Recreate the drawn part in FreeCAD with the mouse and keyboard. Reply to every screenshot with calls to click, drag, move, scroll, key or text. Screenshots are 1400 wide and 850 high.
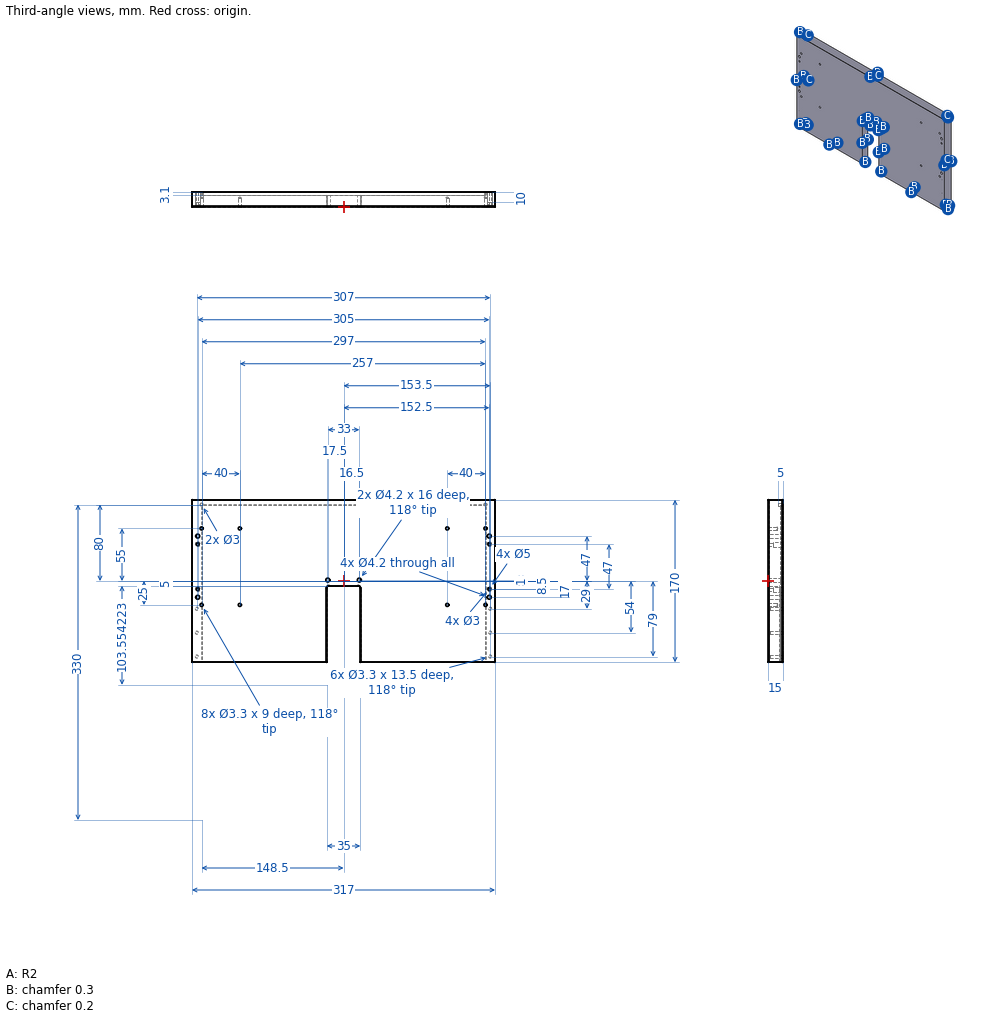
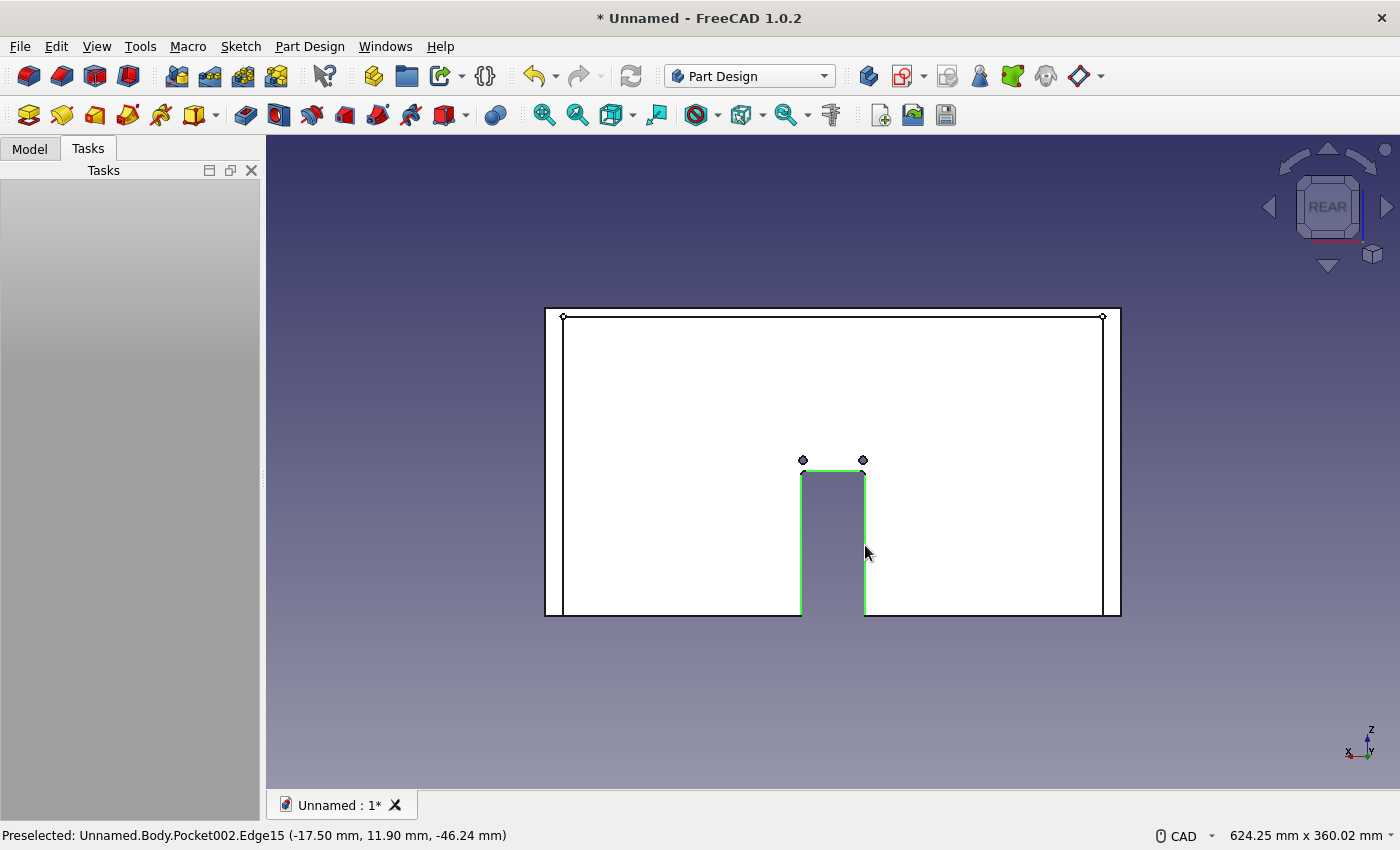
key(6)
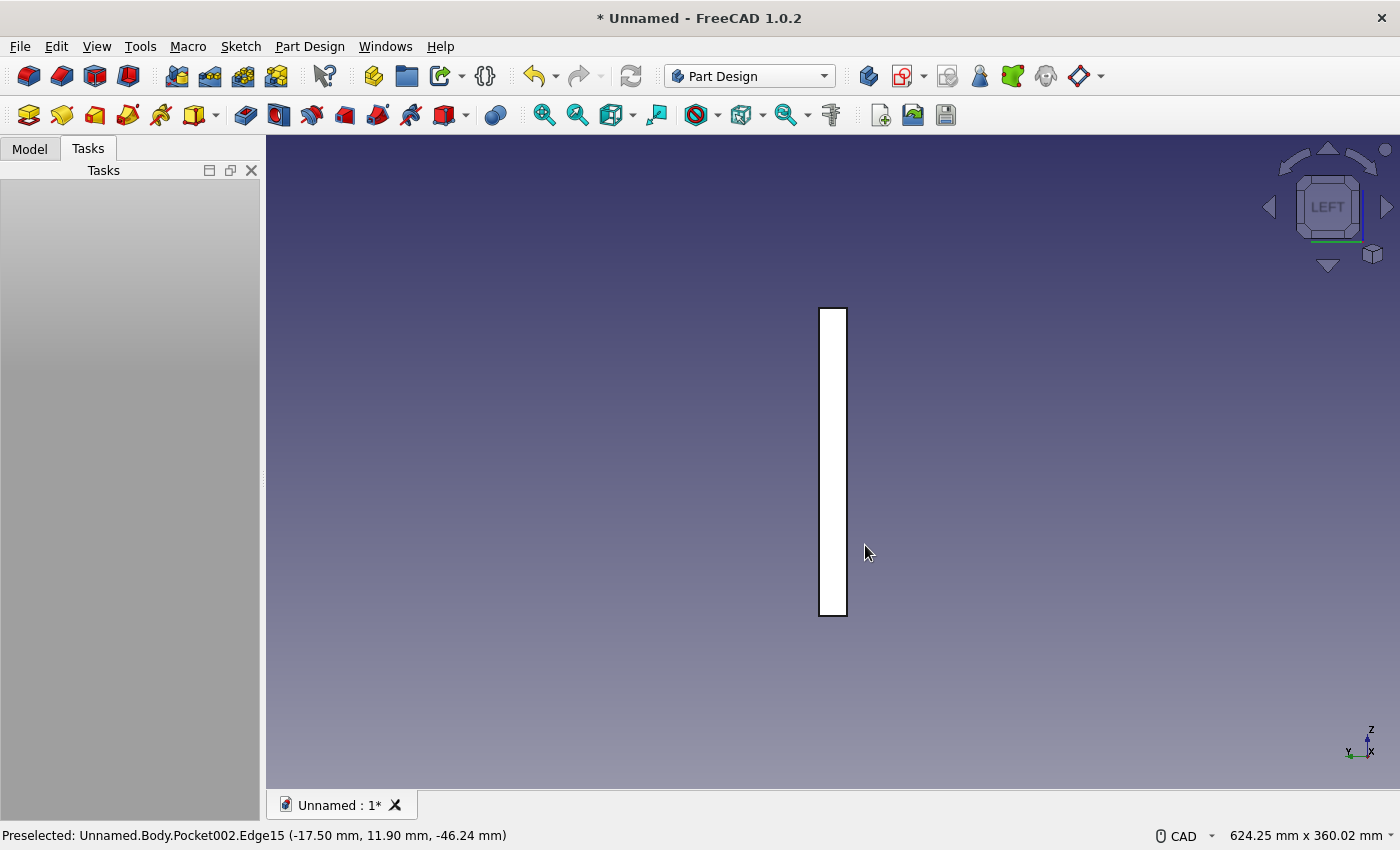
click(833, 329, ctrl)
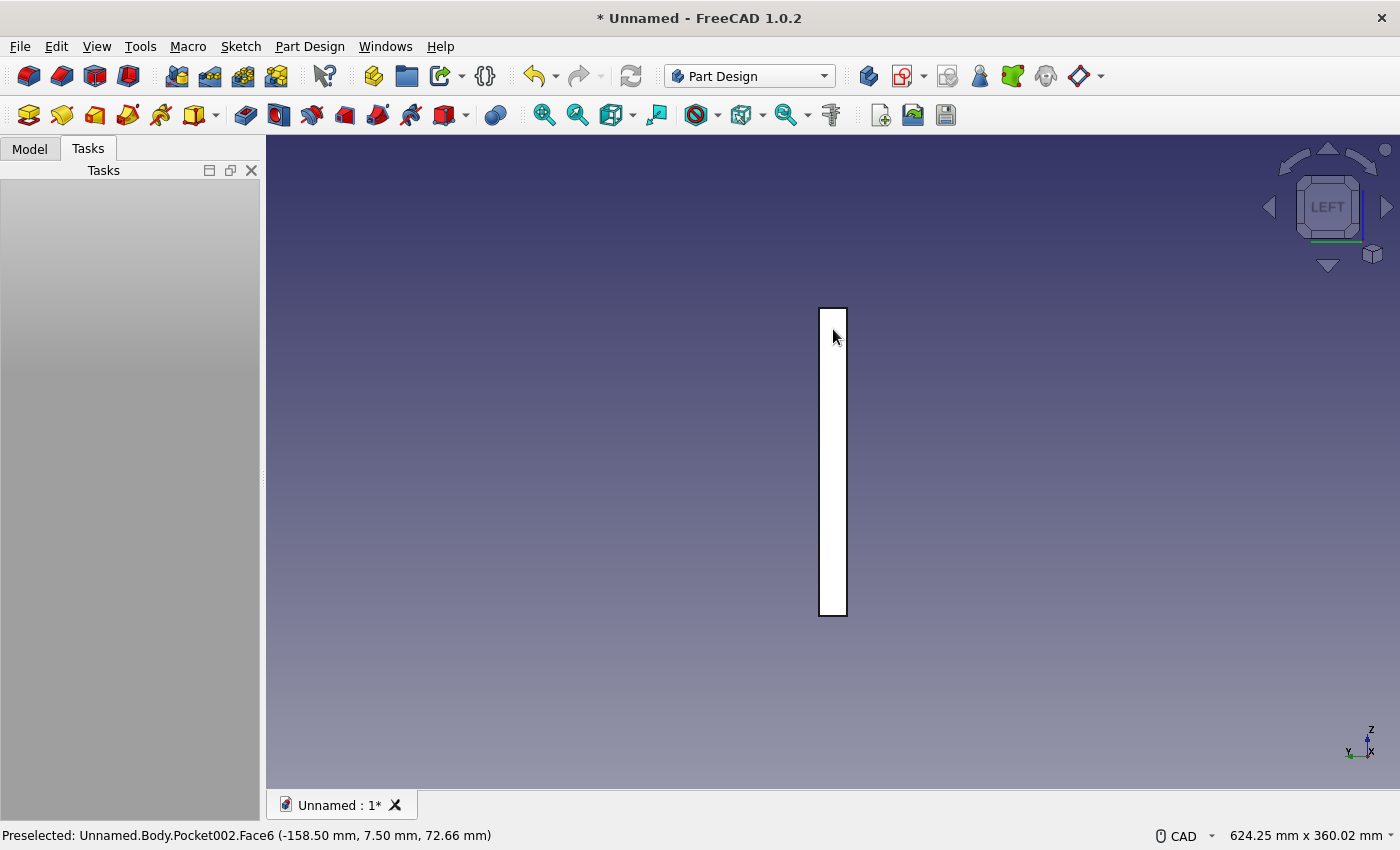
scroll(847, 471, up, 10)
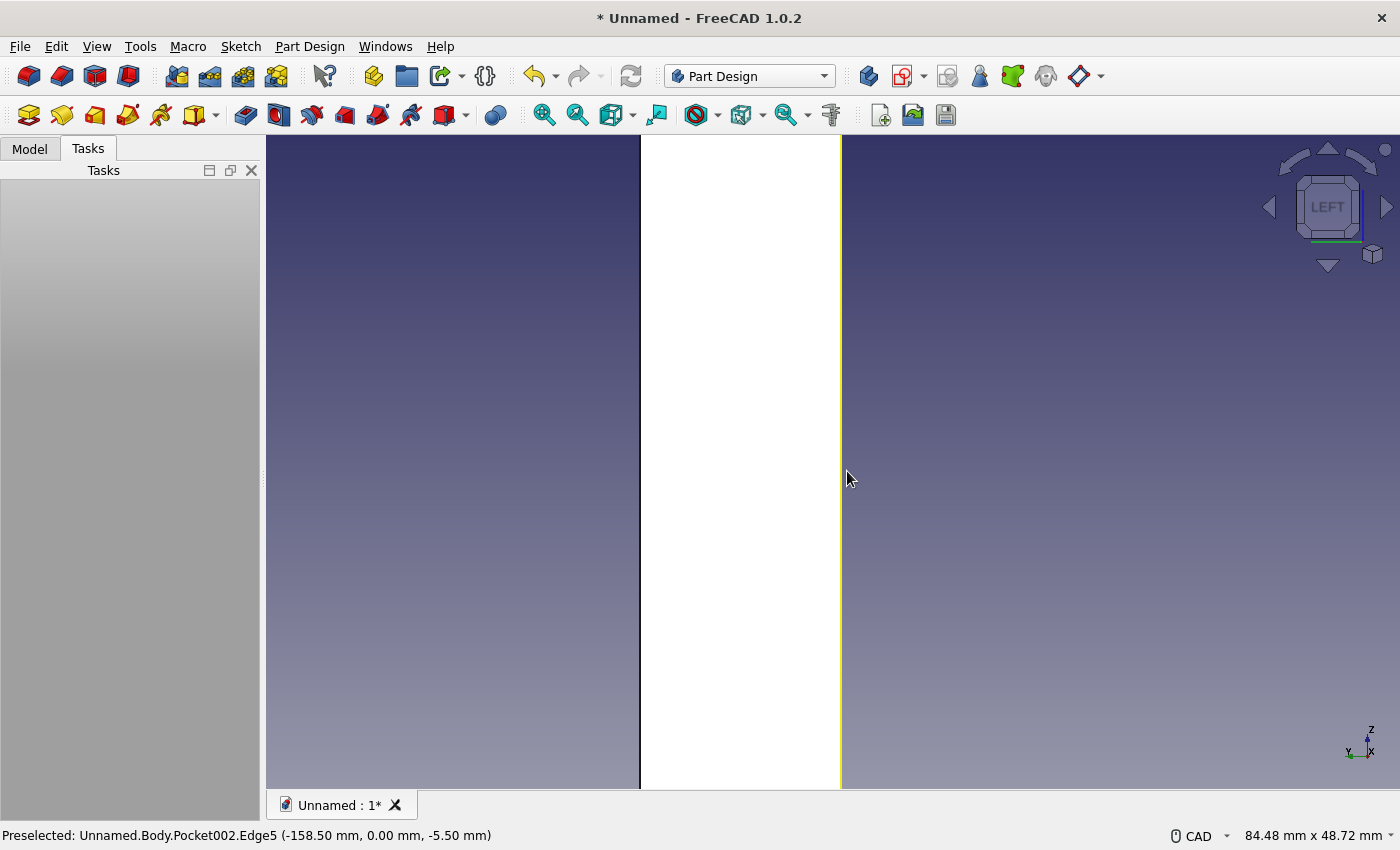
key(v)
key(f)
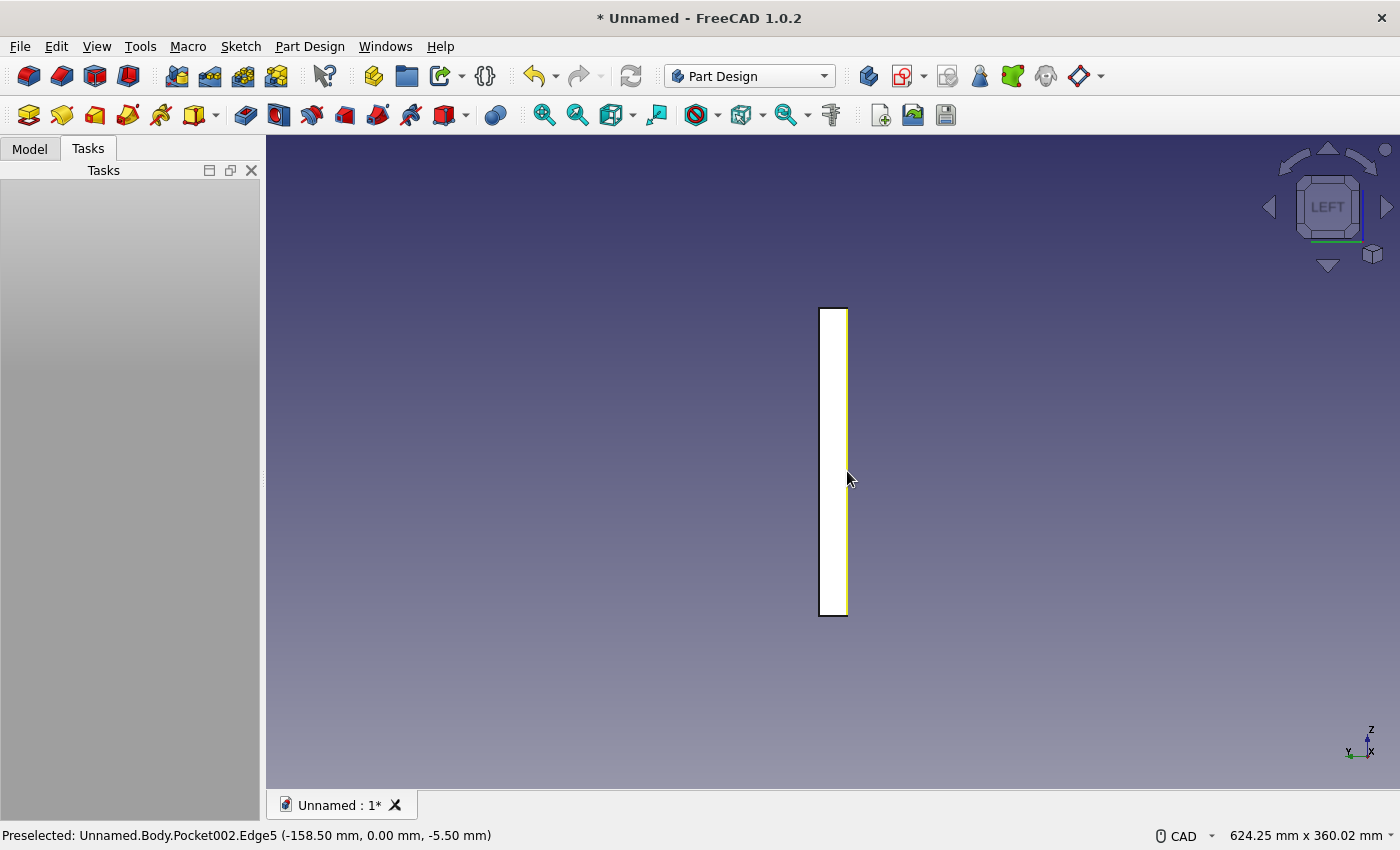
key(v)
key(3)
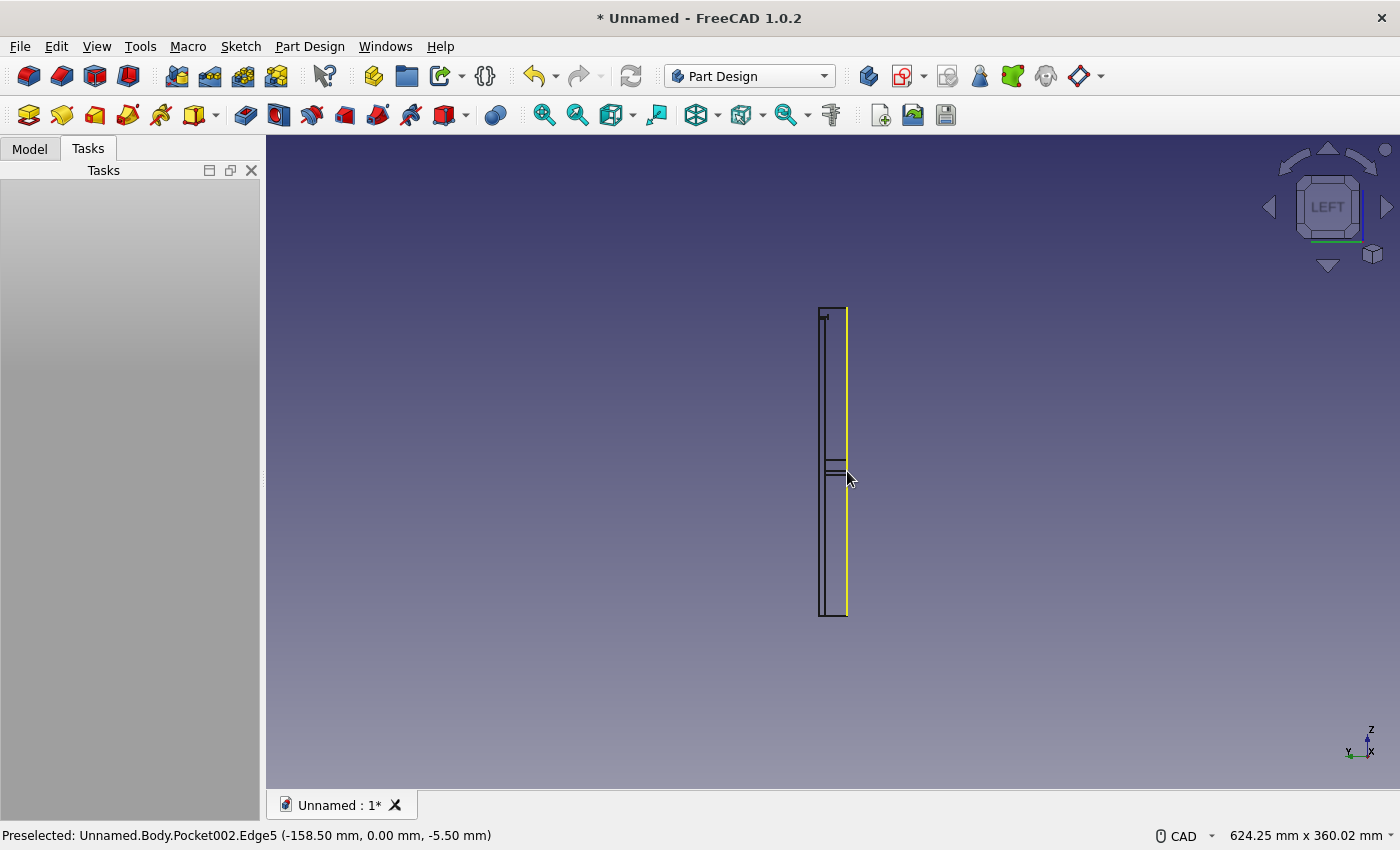
key(0)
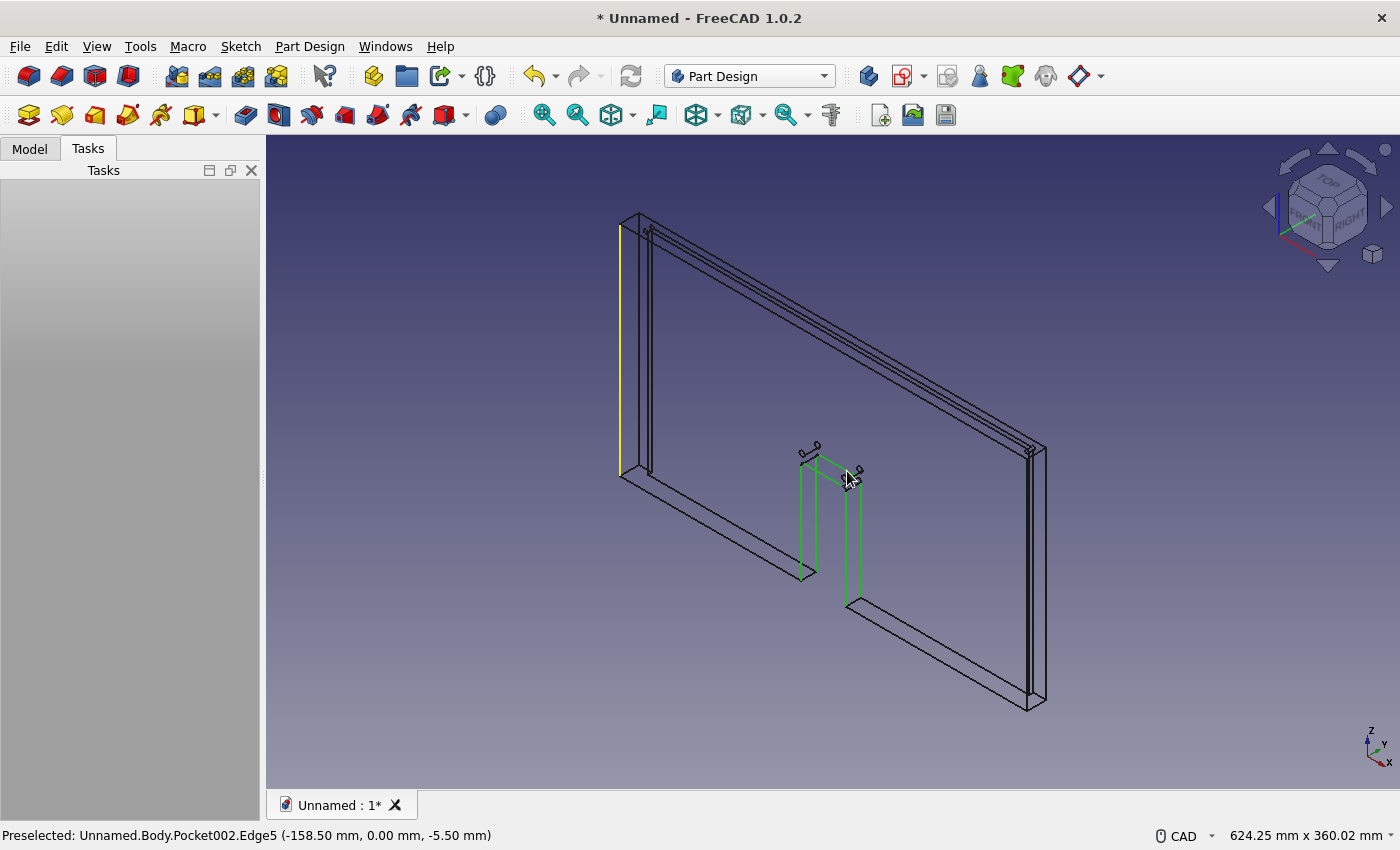
click(845, 487, ctrl)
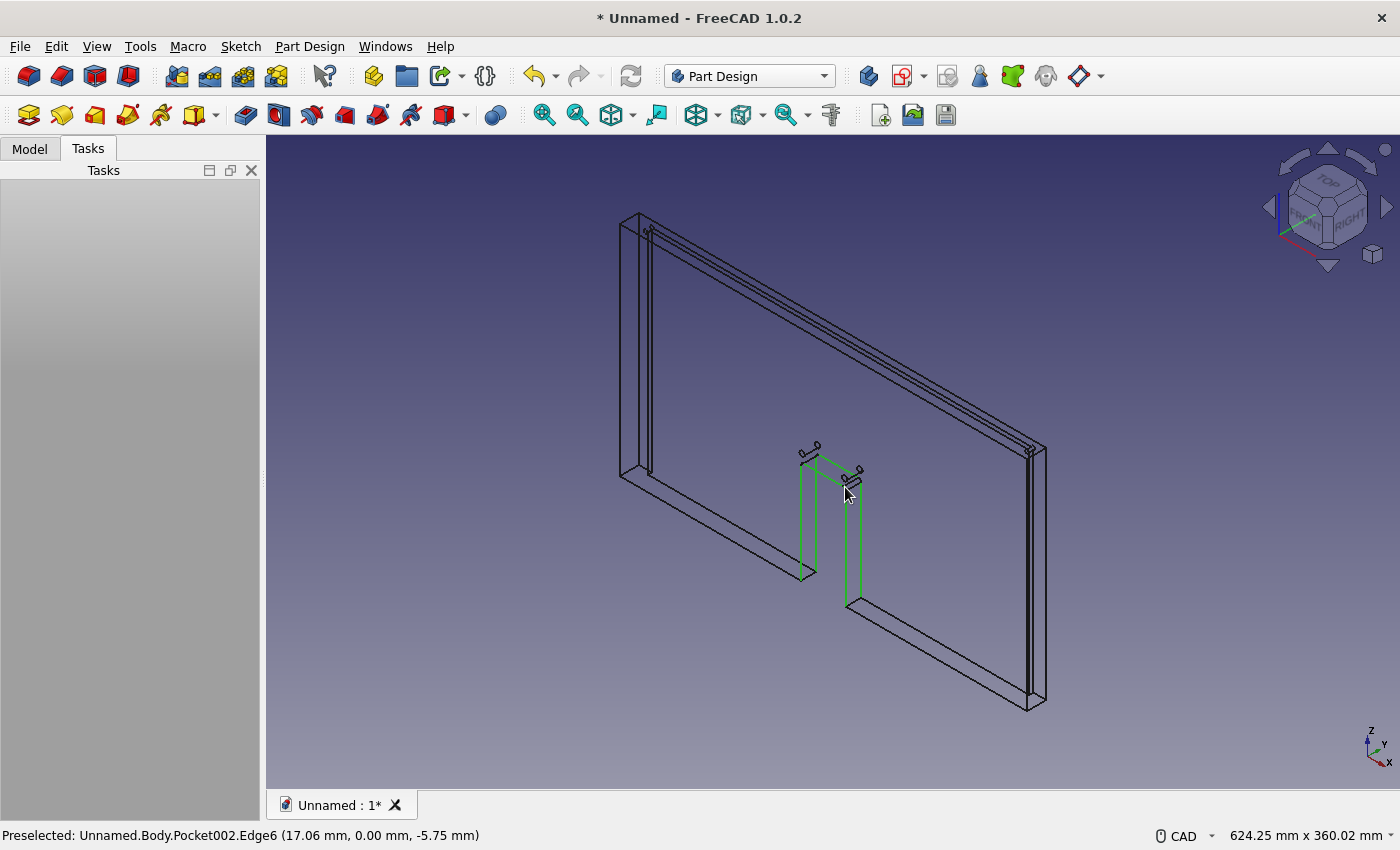
click(861, 479, ctrl)